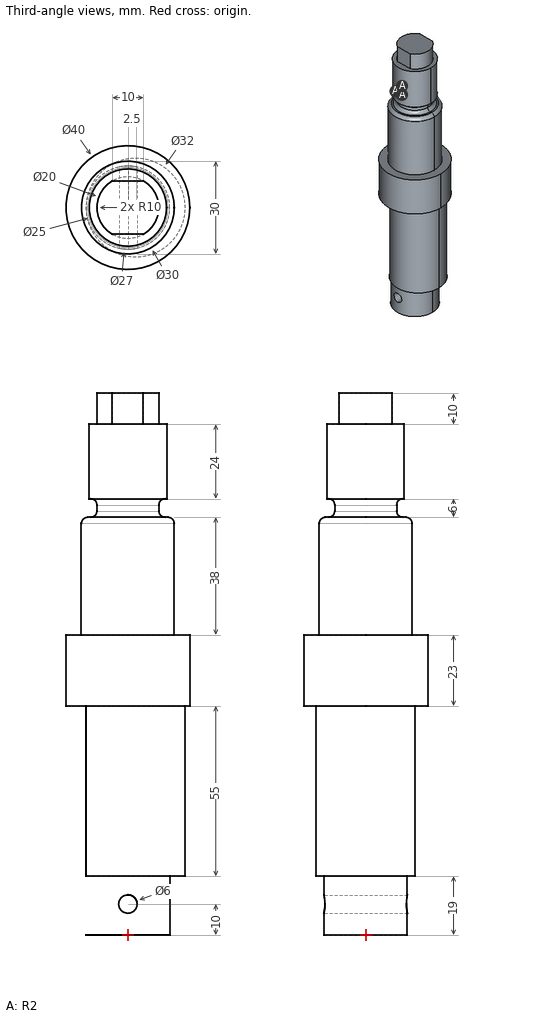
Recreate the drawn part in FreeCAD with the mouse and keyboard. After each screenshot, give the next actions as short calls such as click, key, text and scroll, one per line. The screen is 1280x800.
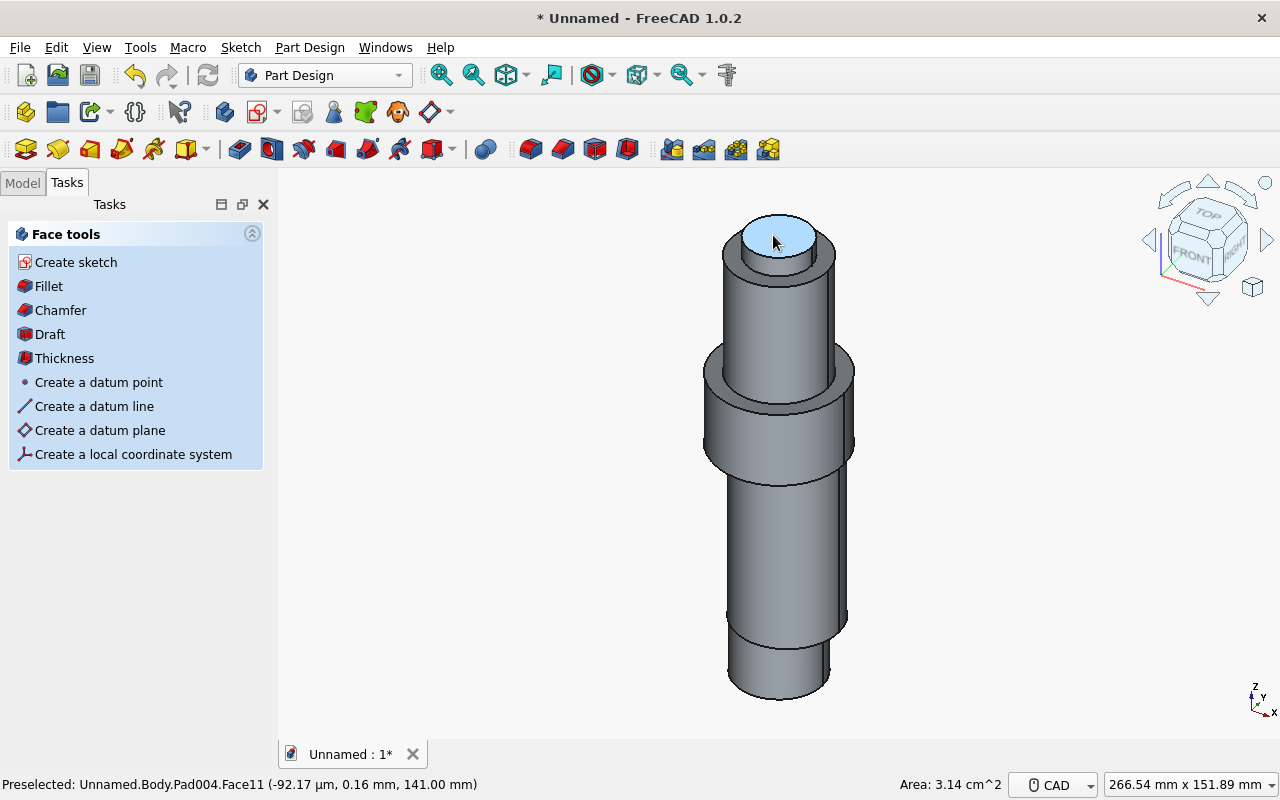
click(258, 112)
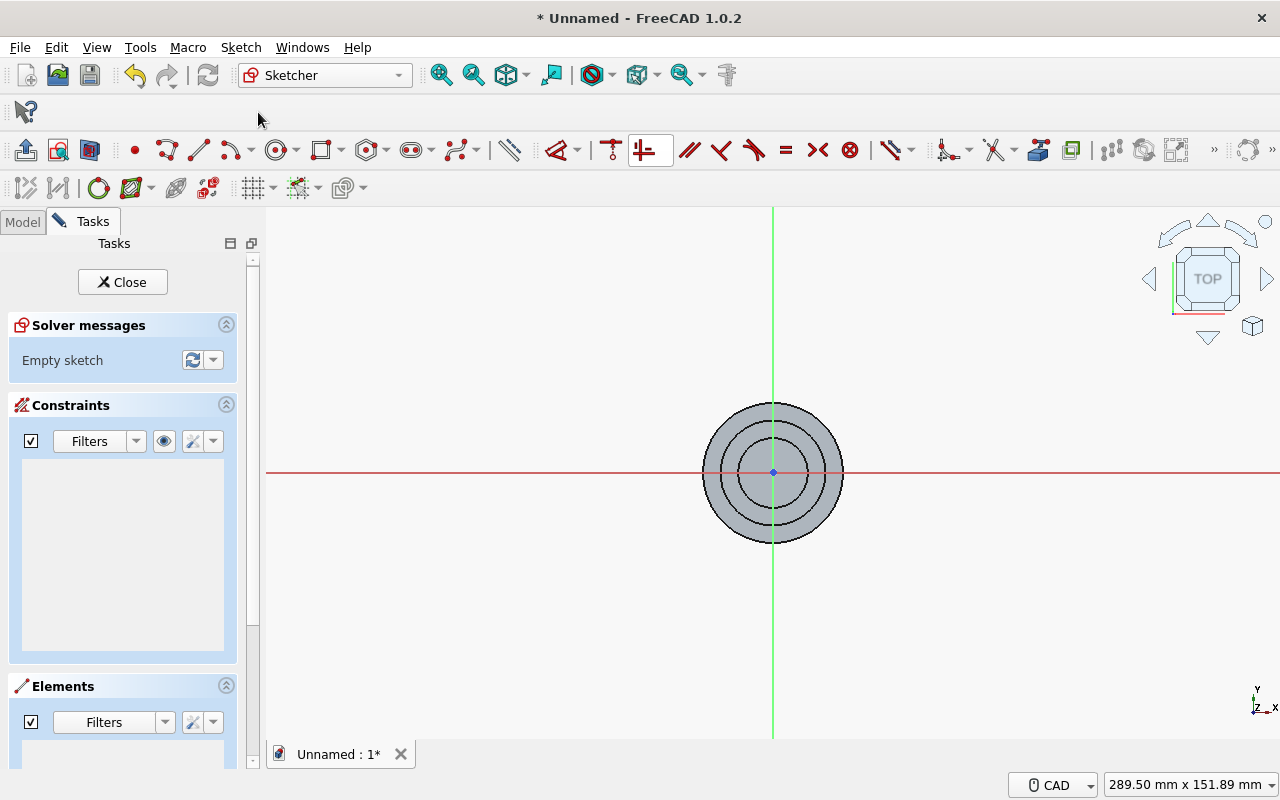
scroll(795, 473, up, 7)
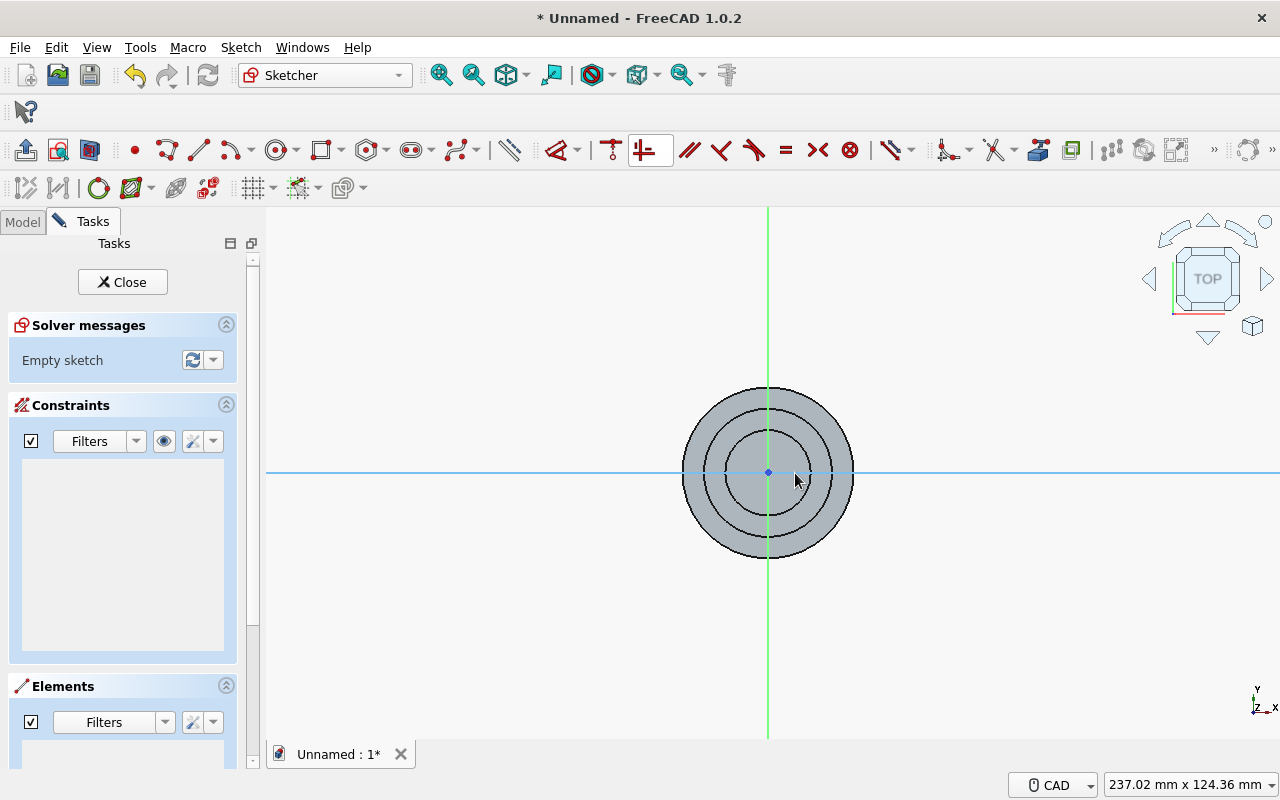
click(276, 150)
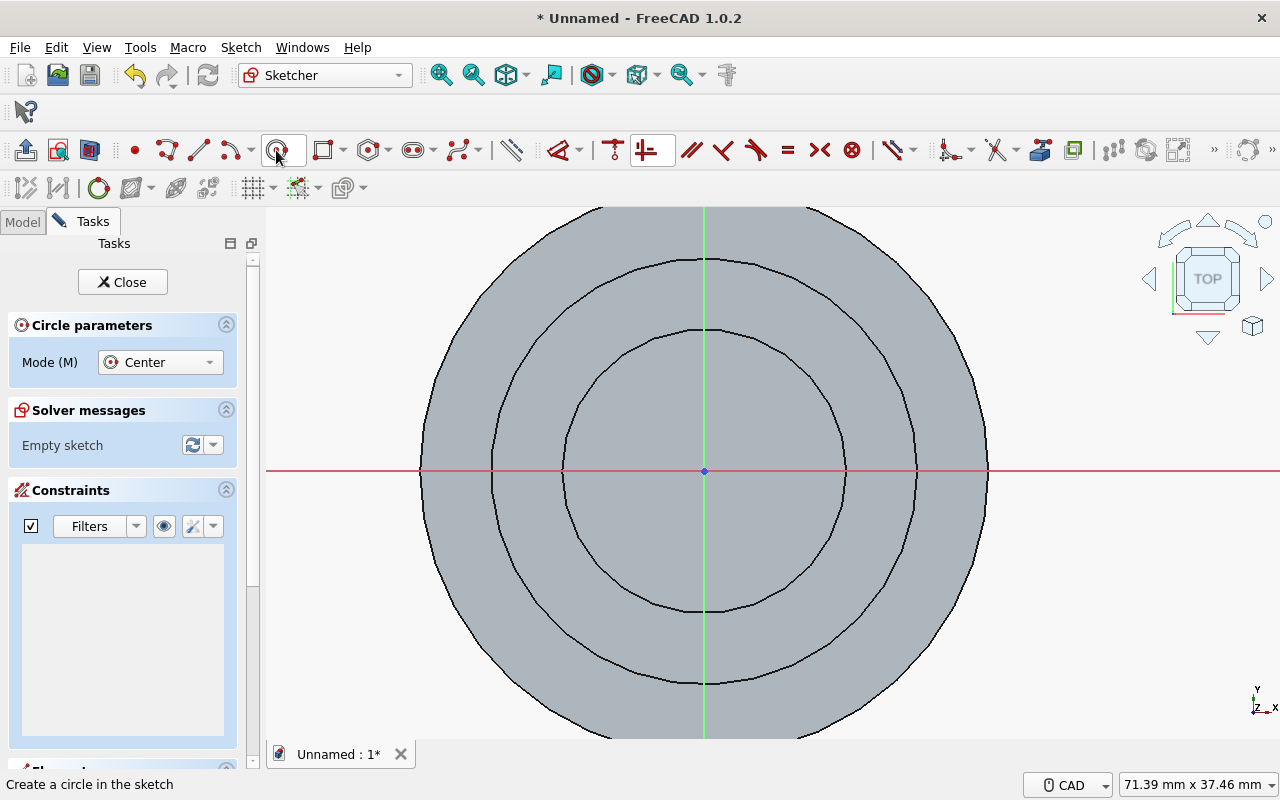
click(704, 471)
click(830, 346)
key(Escape)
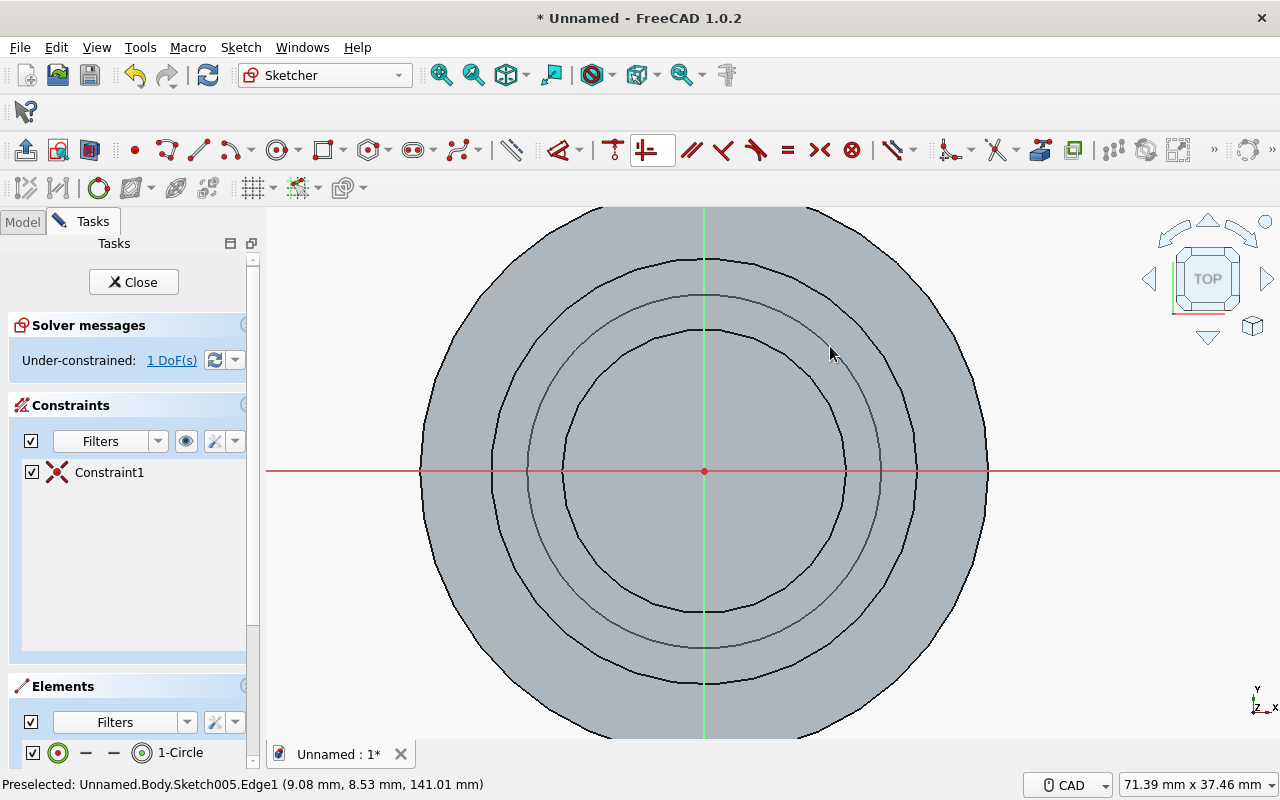
key(d)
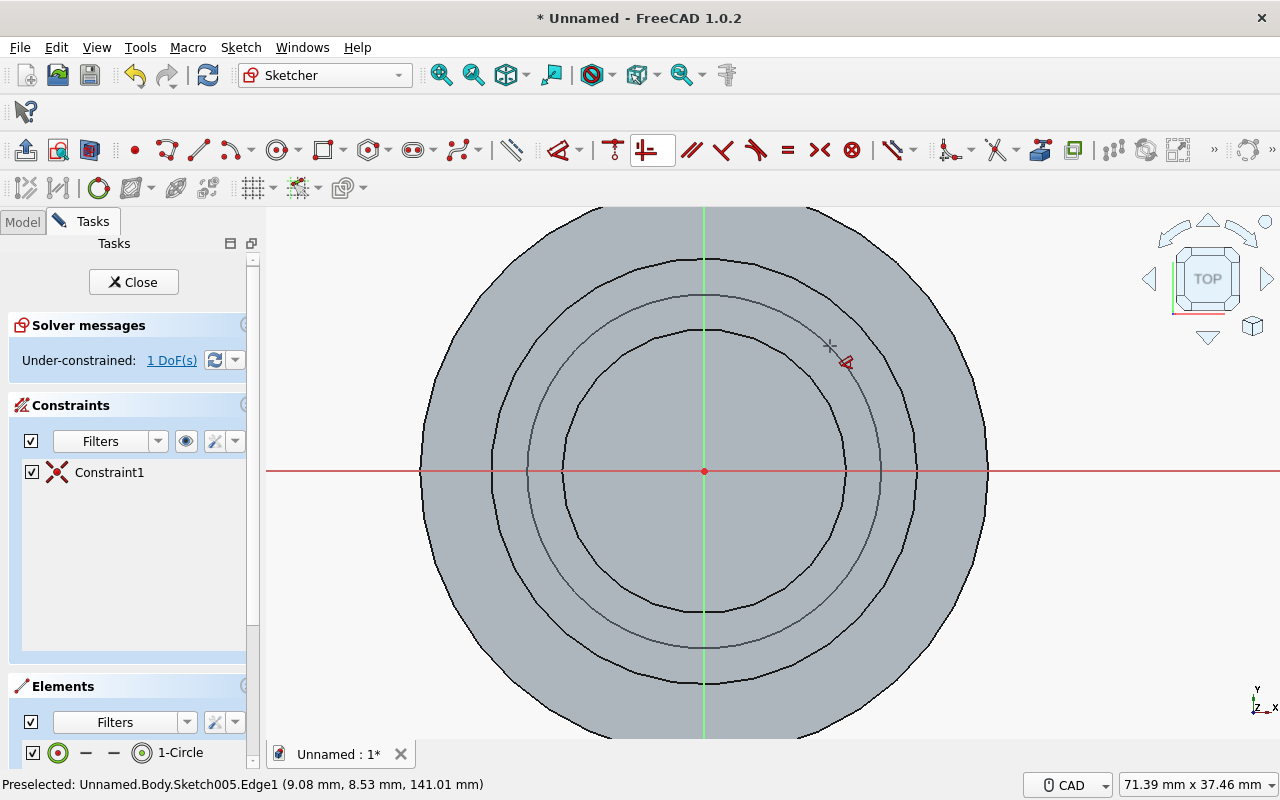
click(829, 346)
click(852, 323)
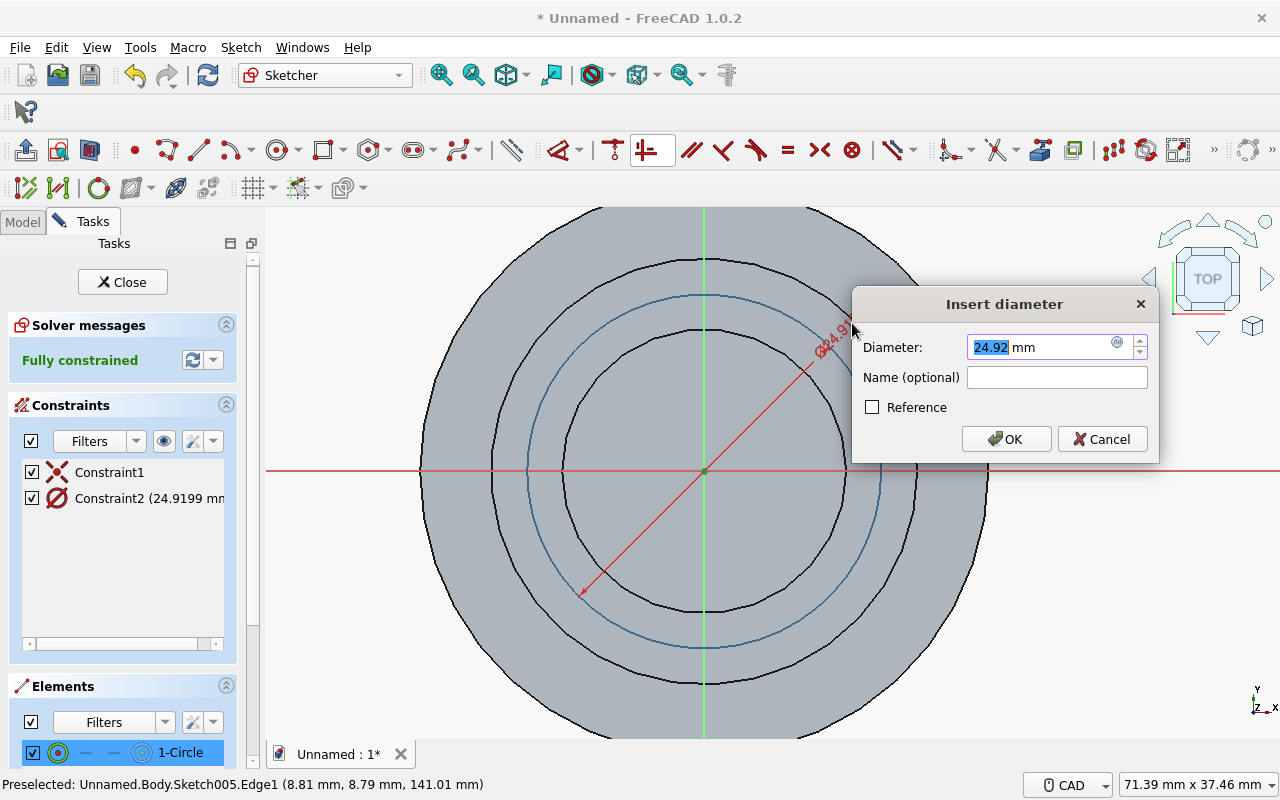
text(25)
key(Return)
key(Escape)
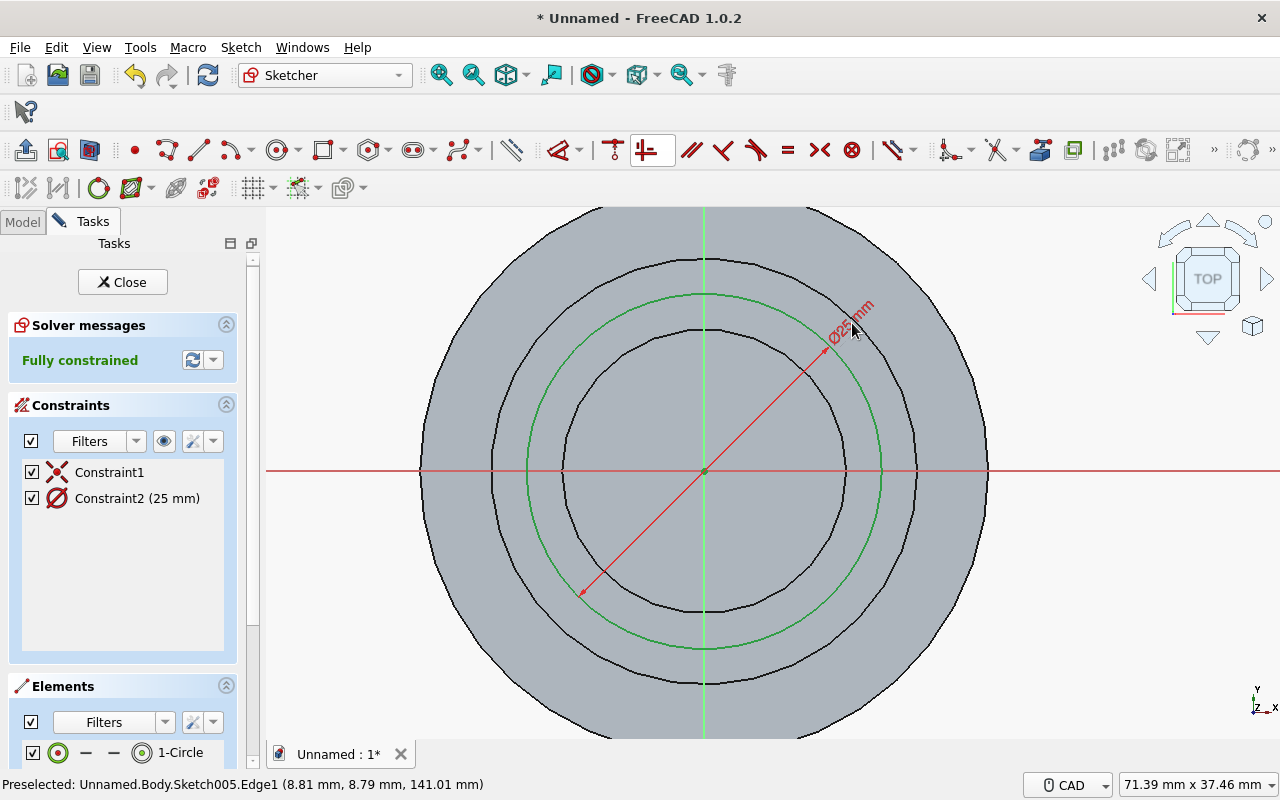
click(123, 282)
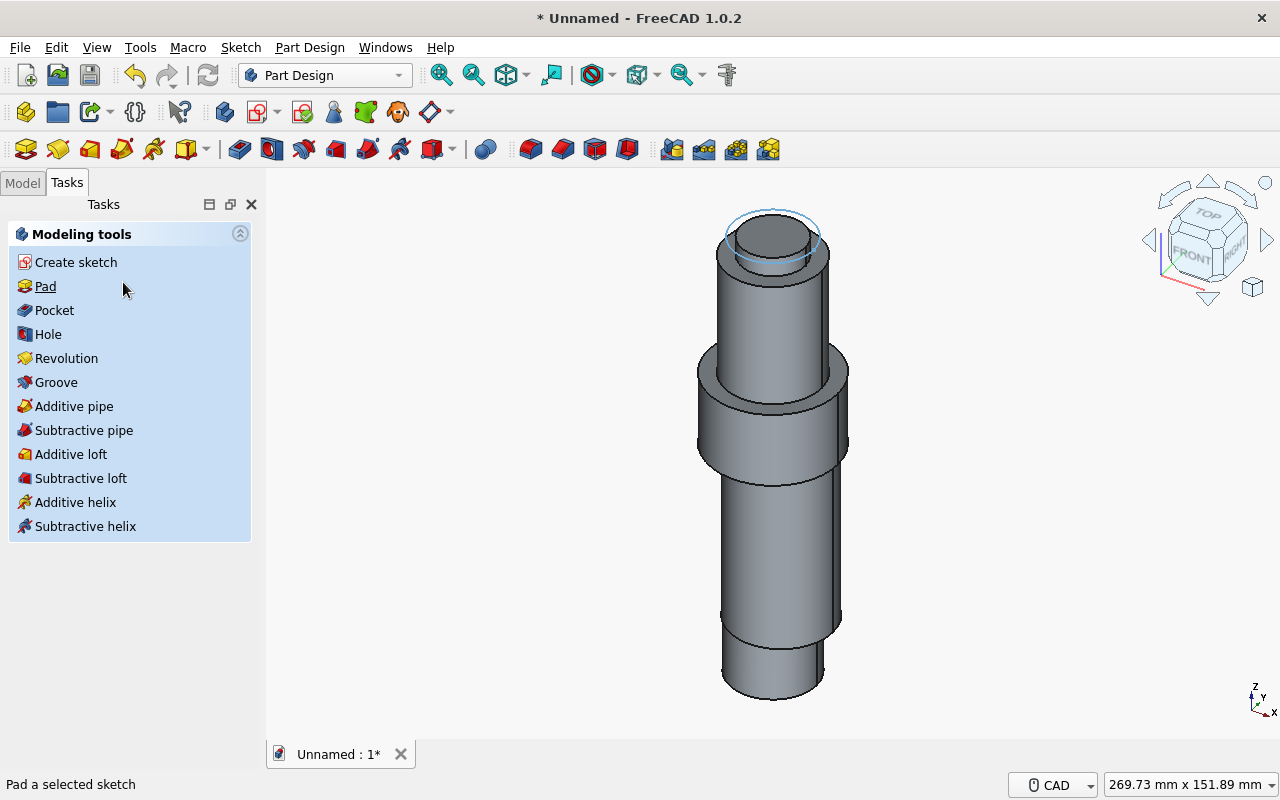
click(26, 150)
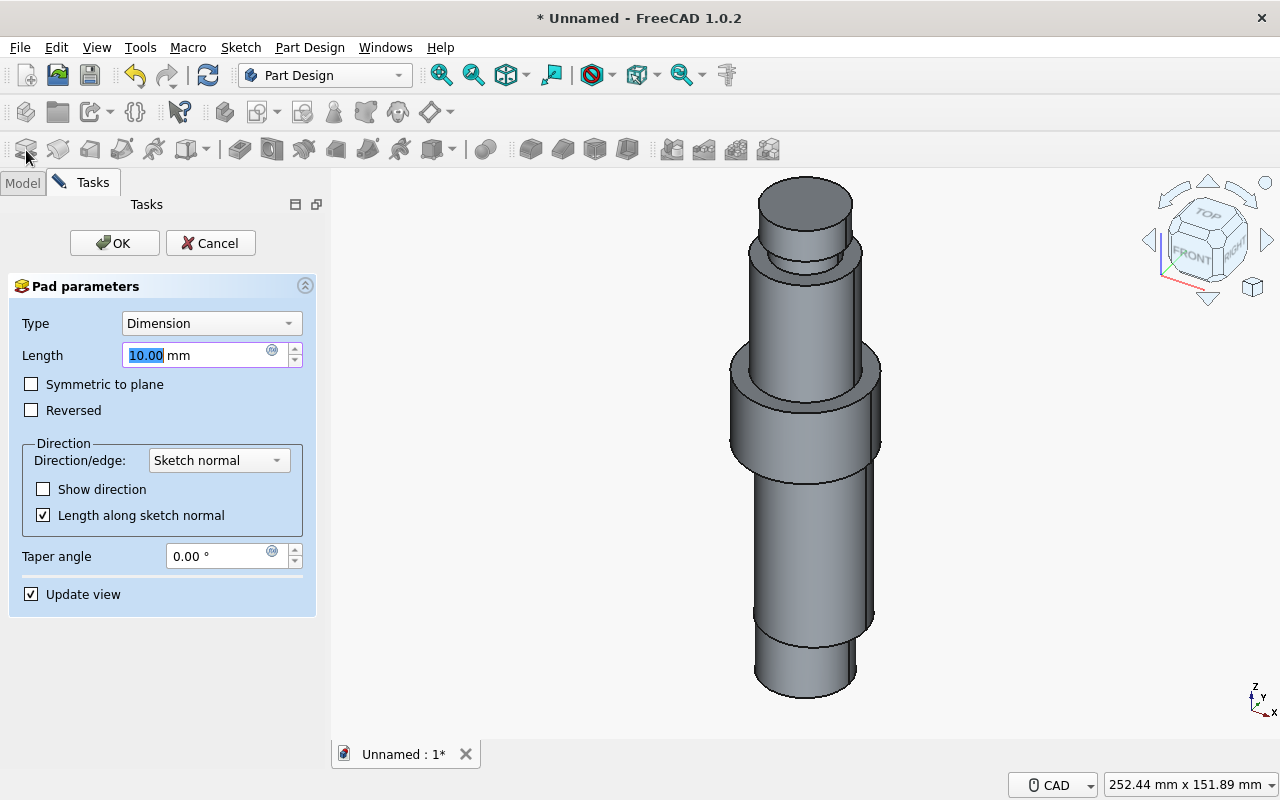
text(24)
key(Tab)